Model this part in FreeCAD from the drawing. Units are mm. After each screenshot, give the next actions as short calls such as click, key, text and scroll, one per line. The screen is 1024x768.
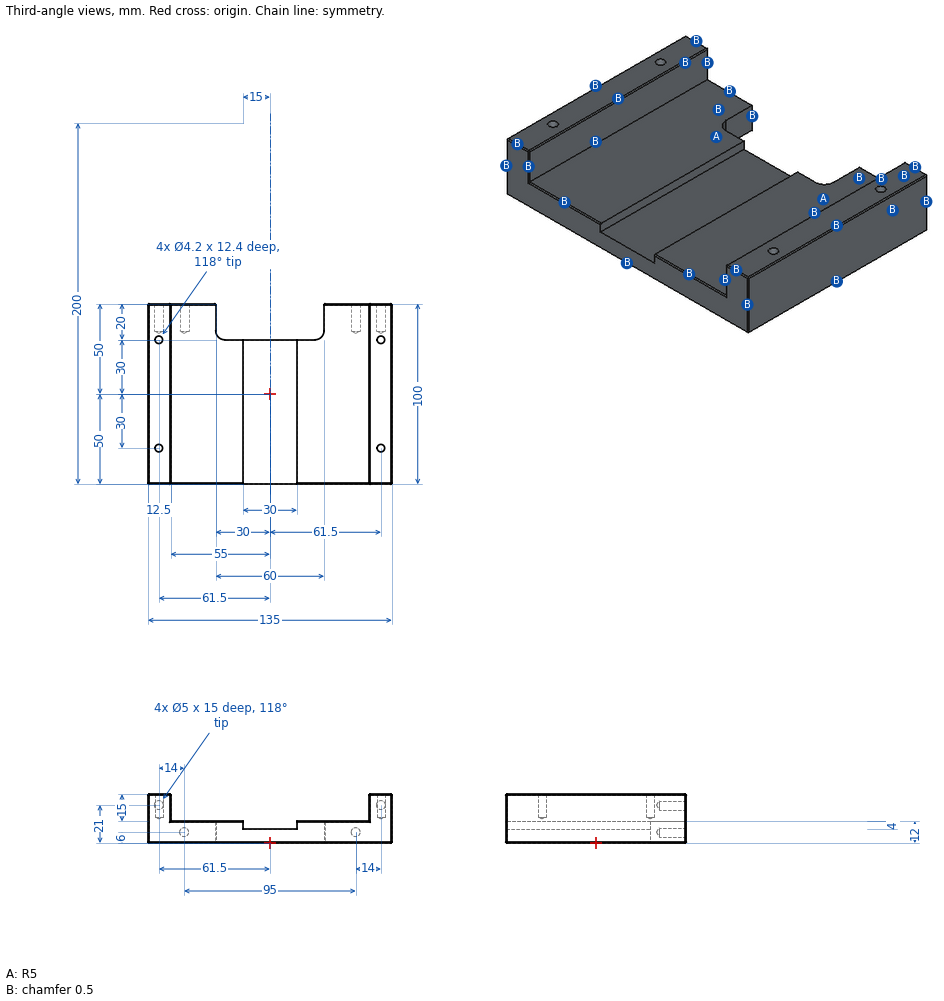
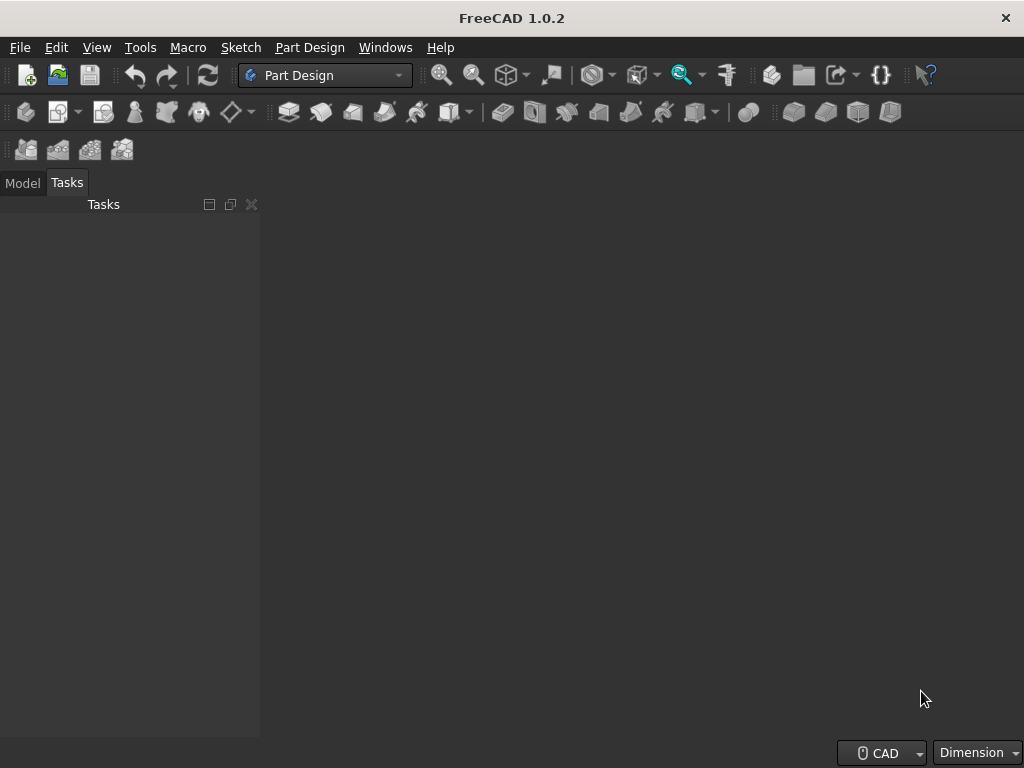
key(ctrl+n)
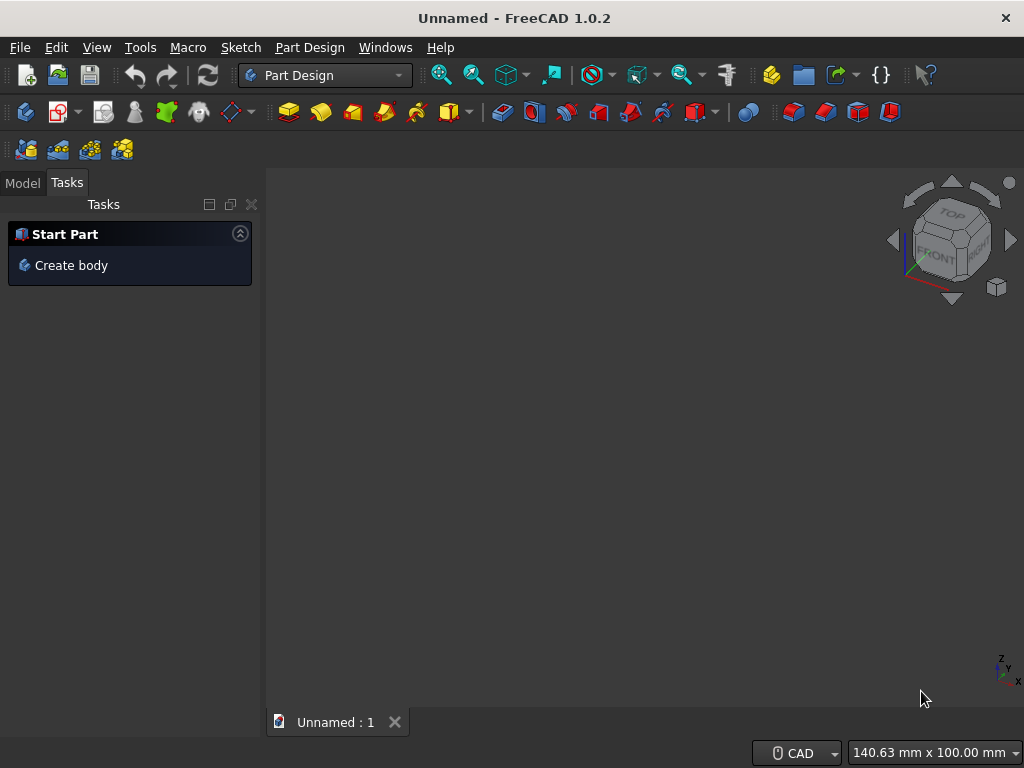
click(58, 112)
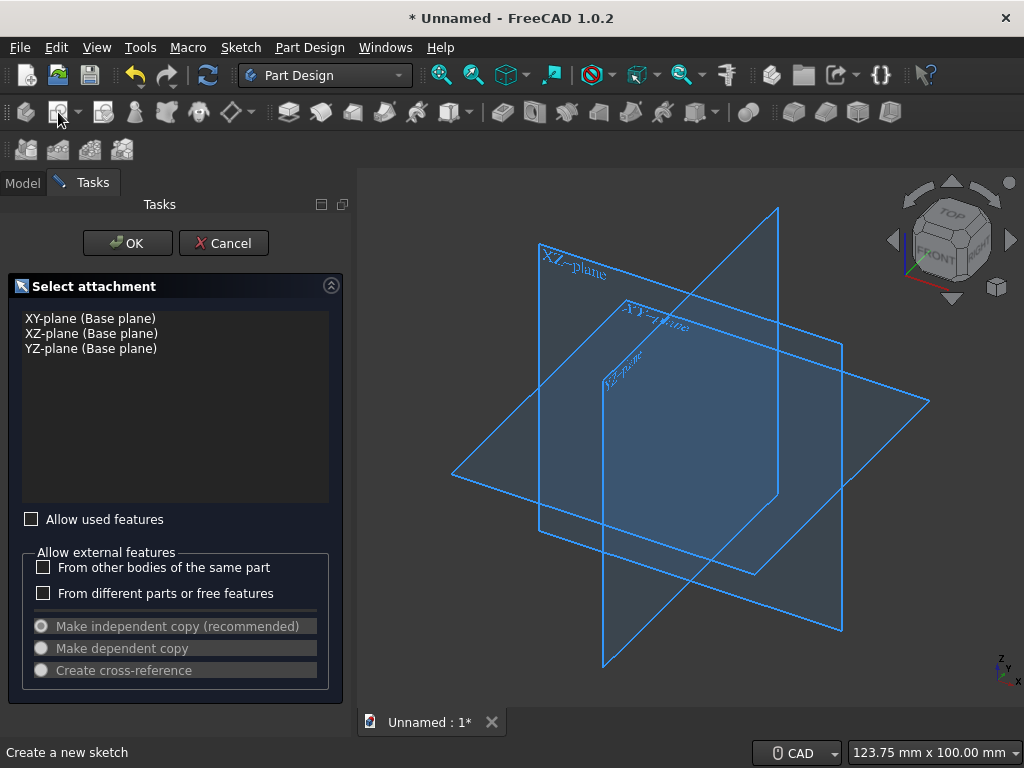
click(82, 318)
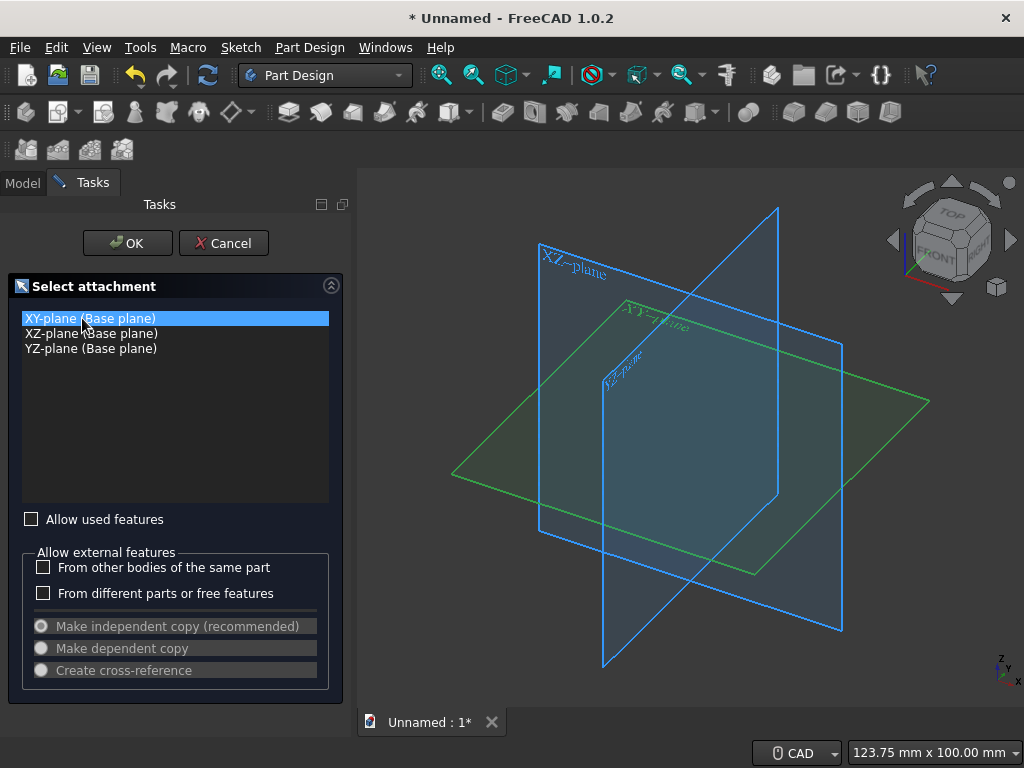
click(128, 243)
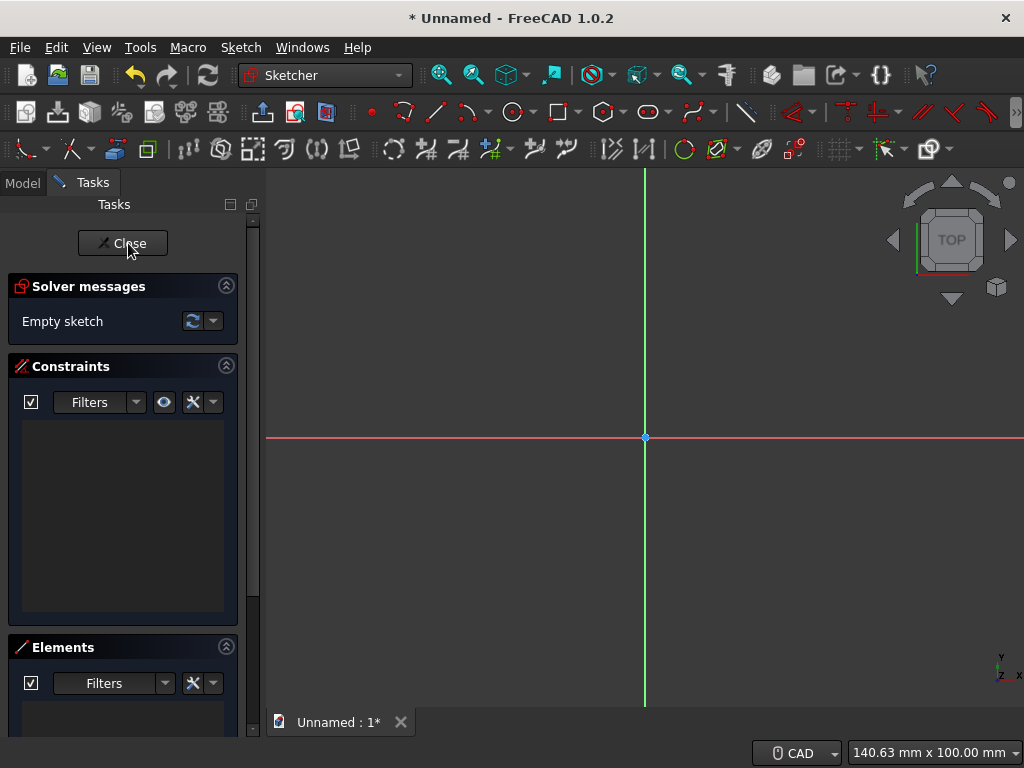
scroll(493, 438, down, 3)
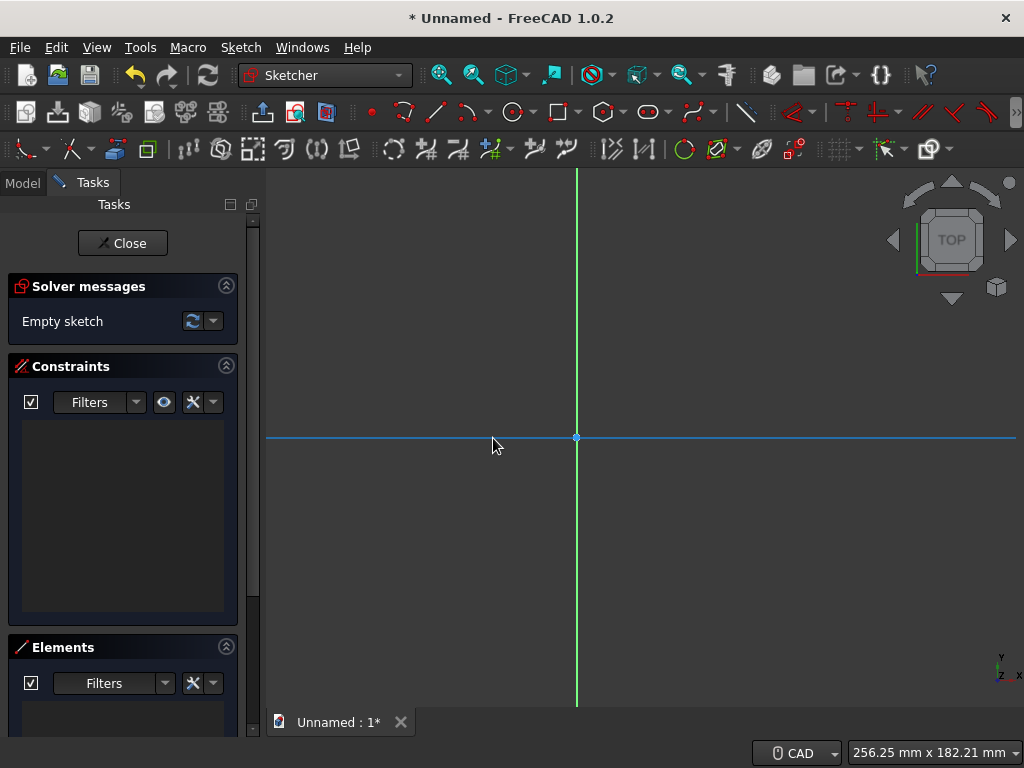
key(g)
key(v)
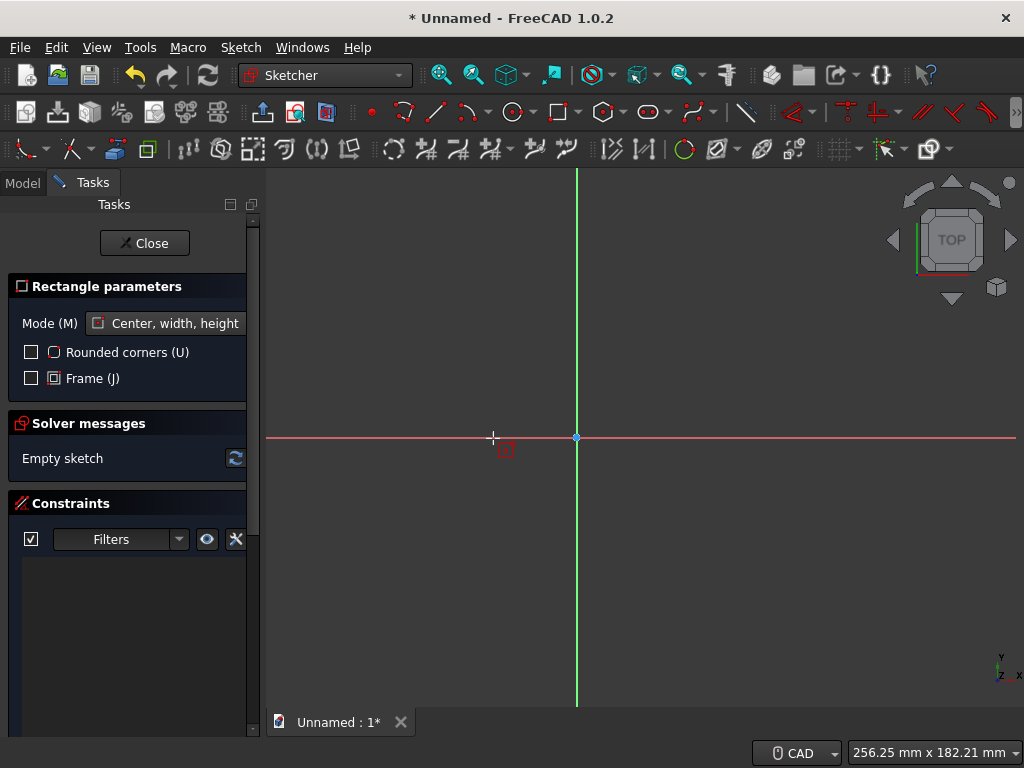
click(577, 438)
click(776, 290)
key(Escape)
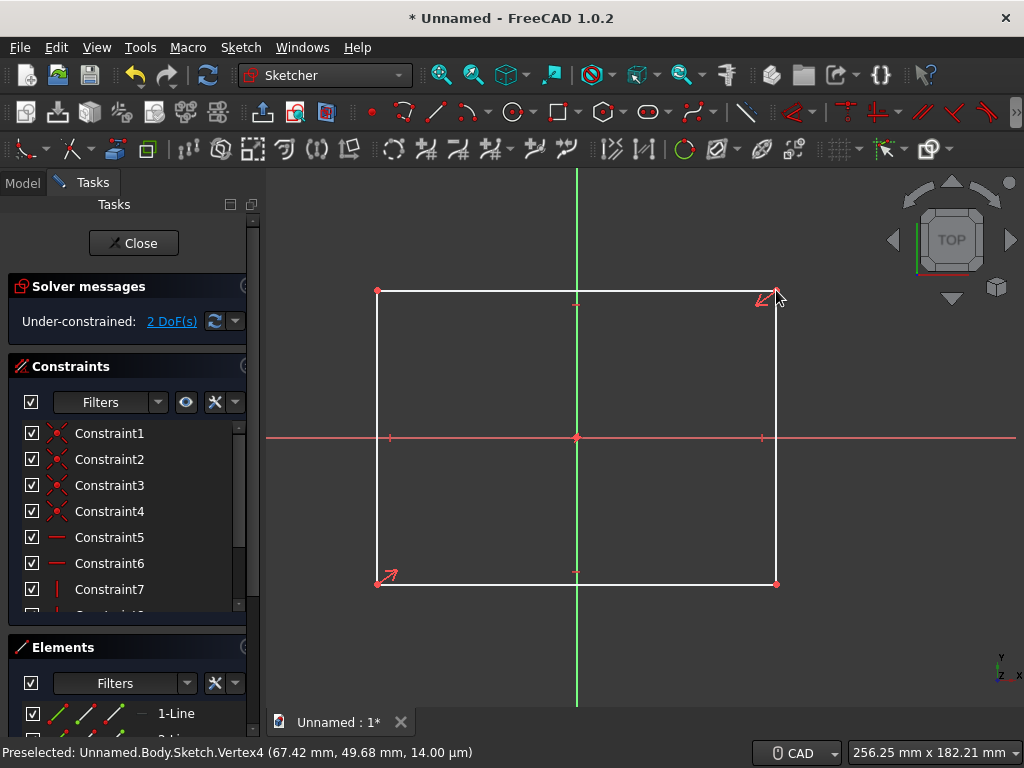
key(d)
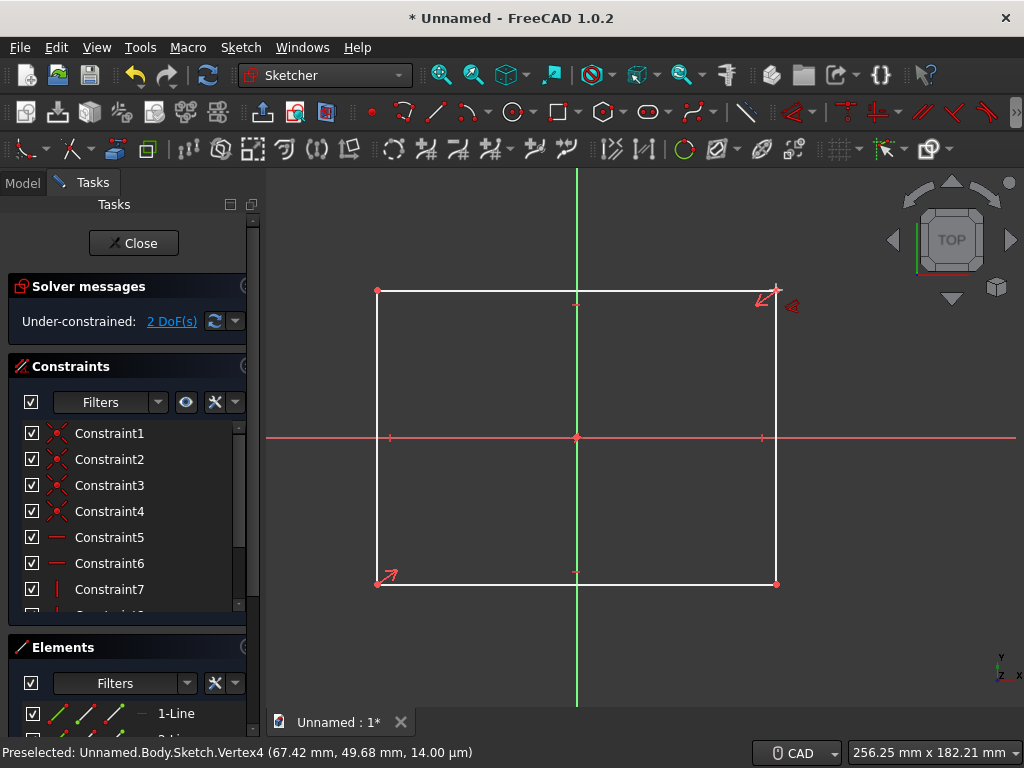
click(497, 585)
click(485, 619)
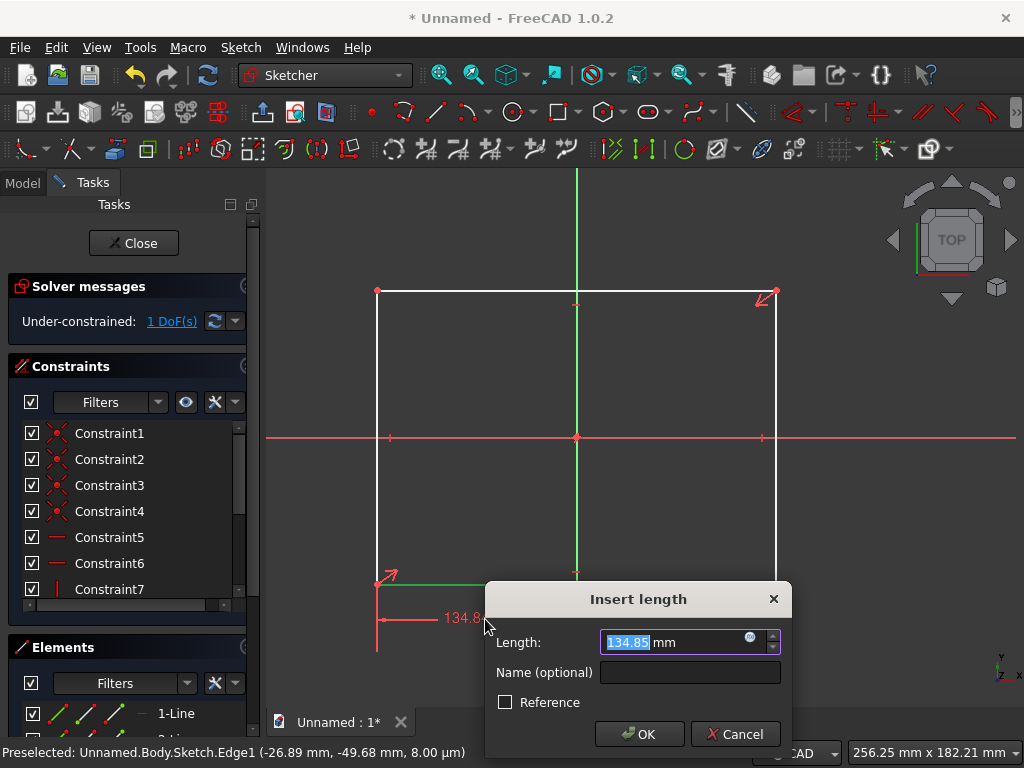
text(135)
key(Return)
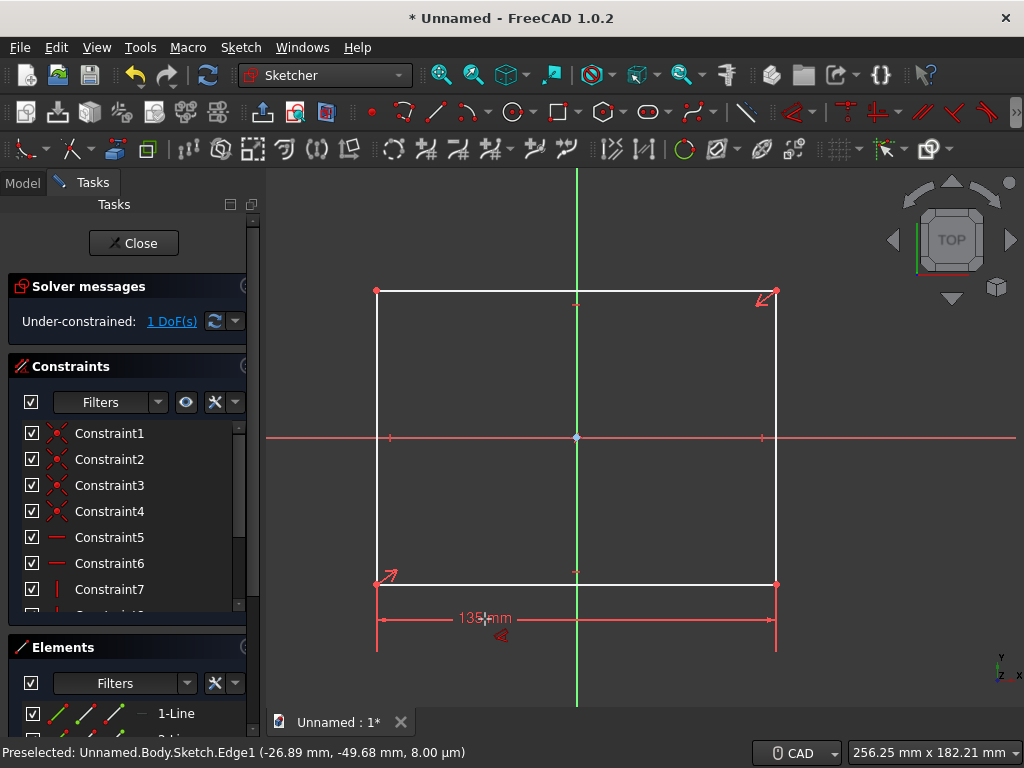
click(776, 497)
click(810, 370)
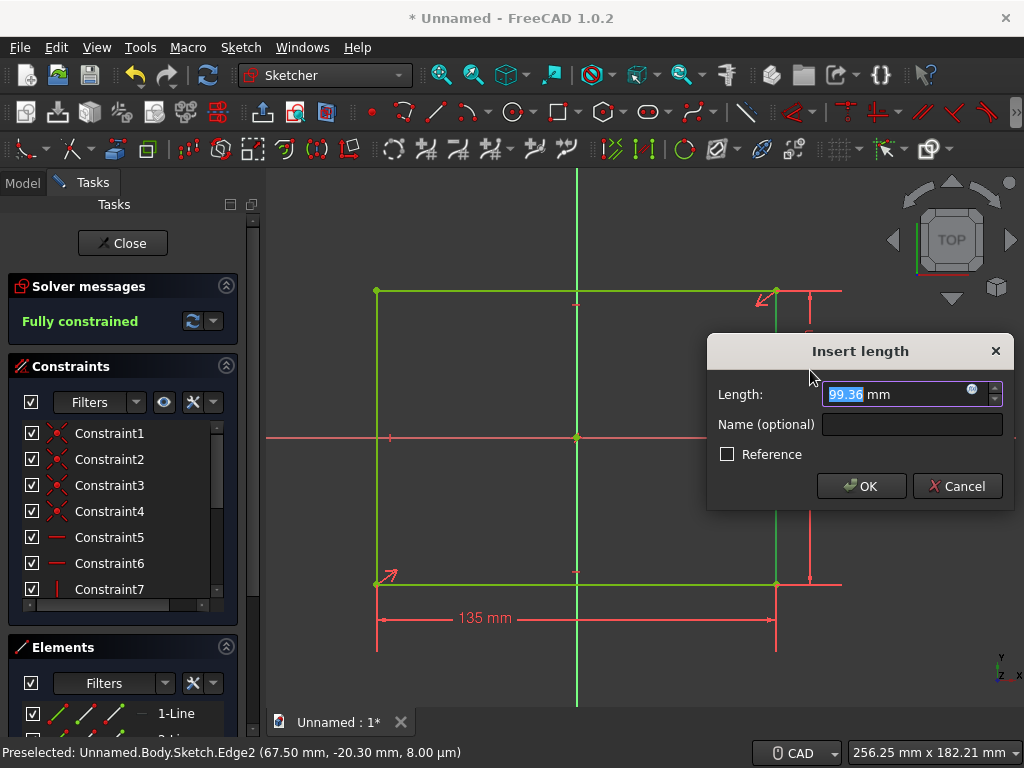
text(100)
key(Return)
key(Escape)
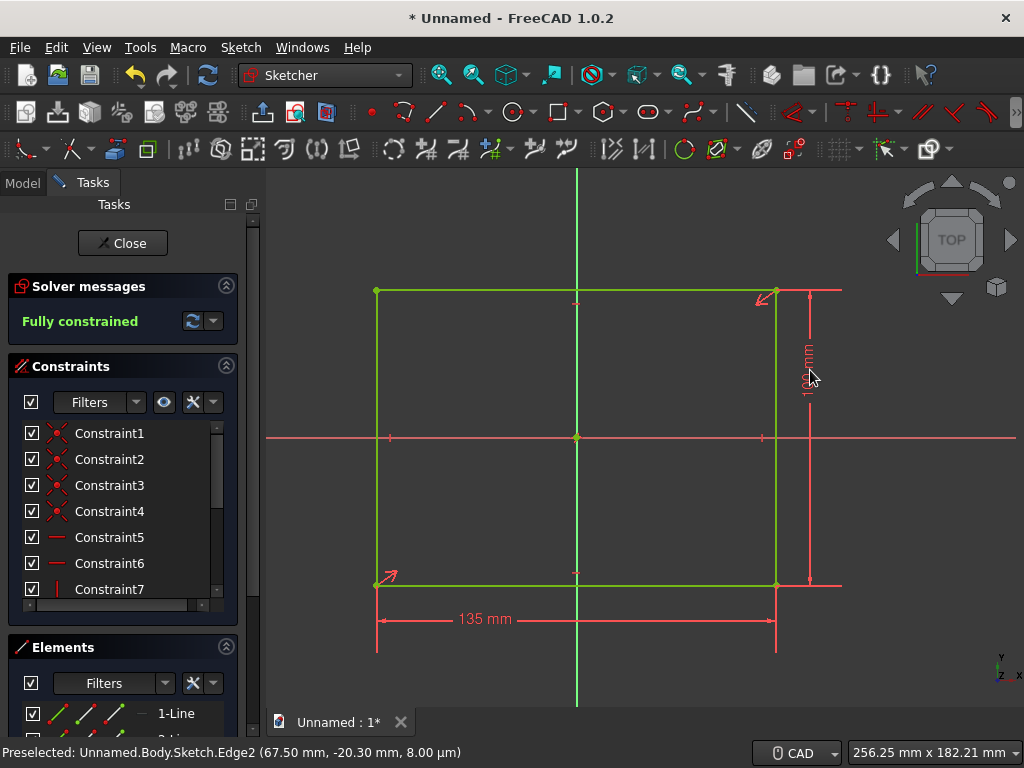
click(123, 243)